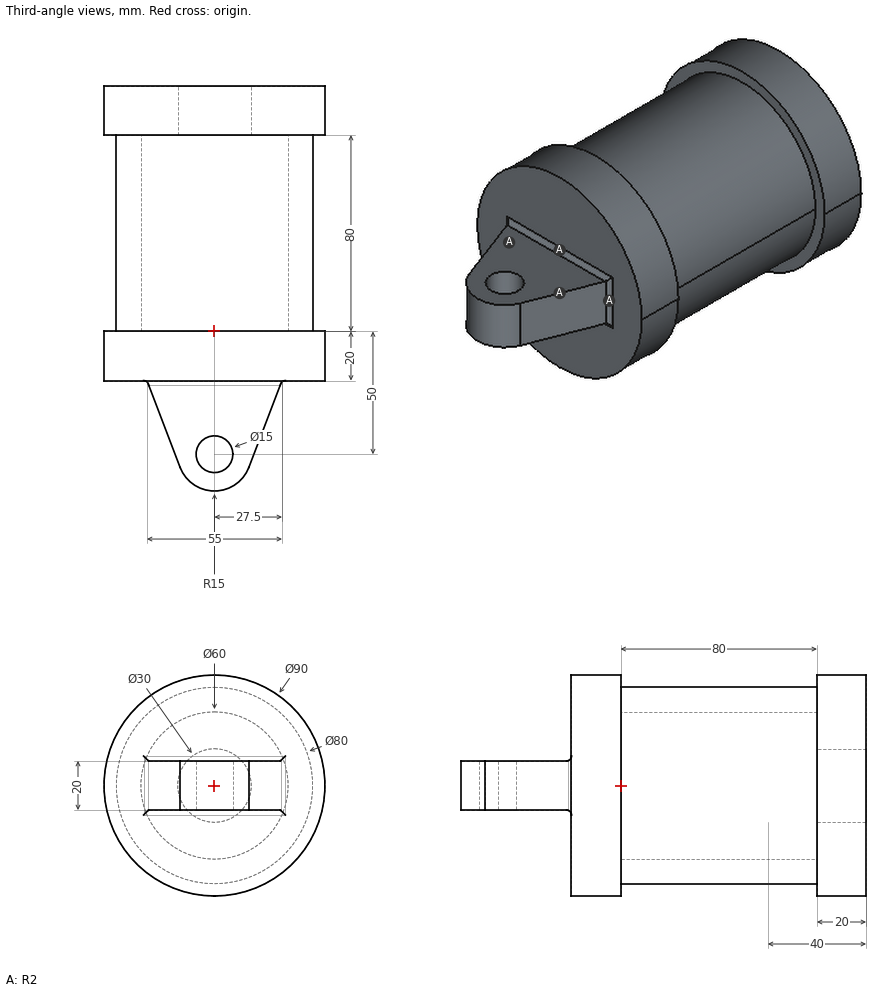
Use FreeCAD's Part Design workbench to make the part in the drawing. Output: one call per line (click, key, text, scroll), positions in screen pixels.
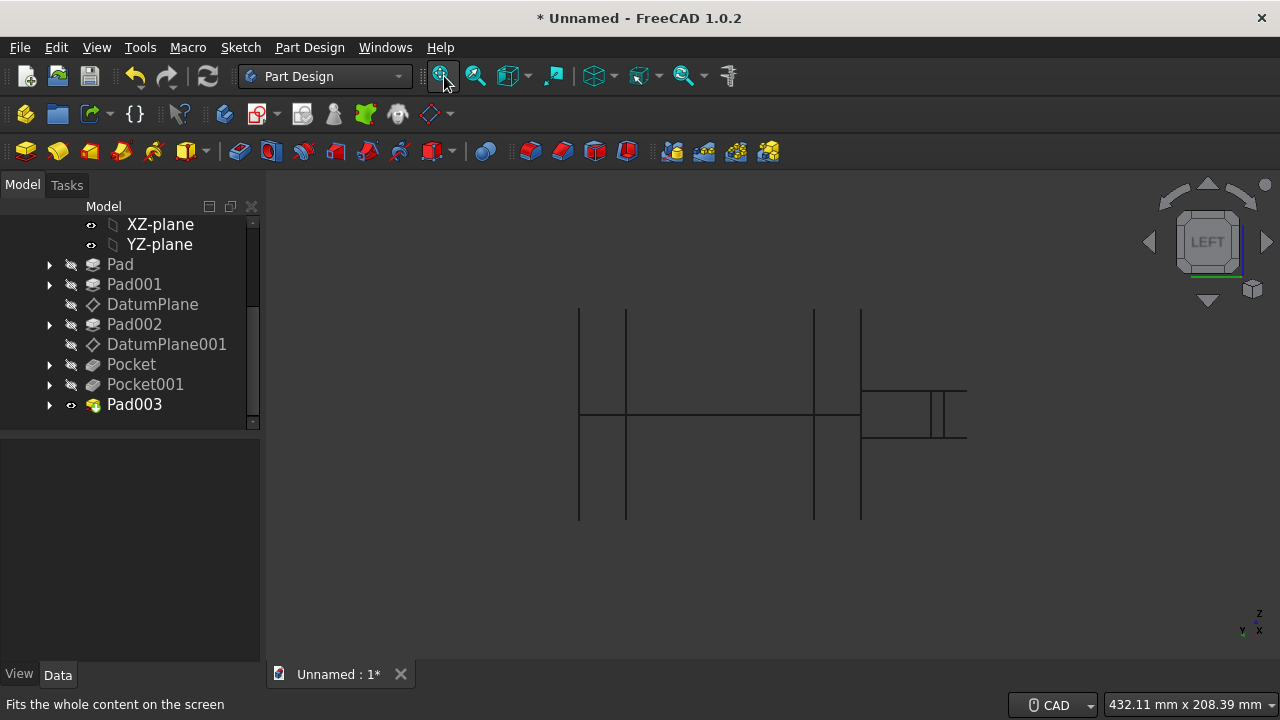
key(0)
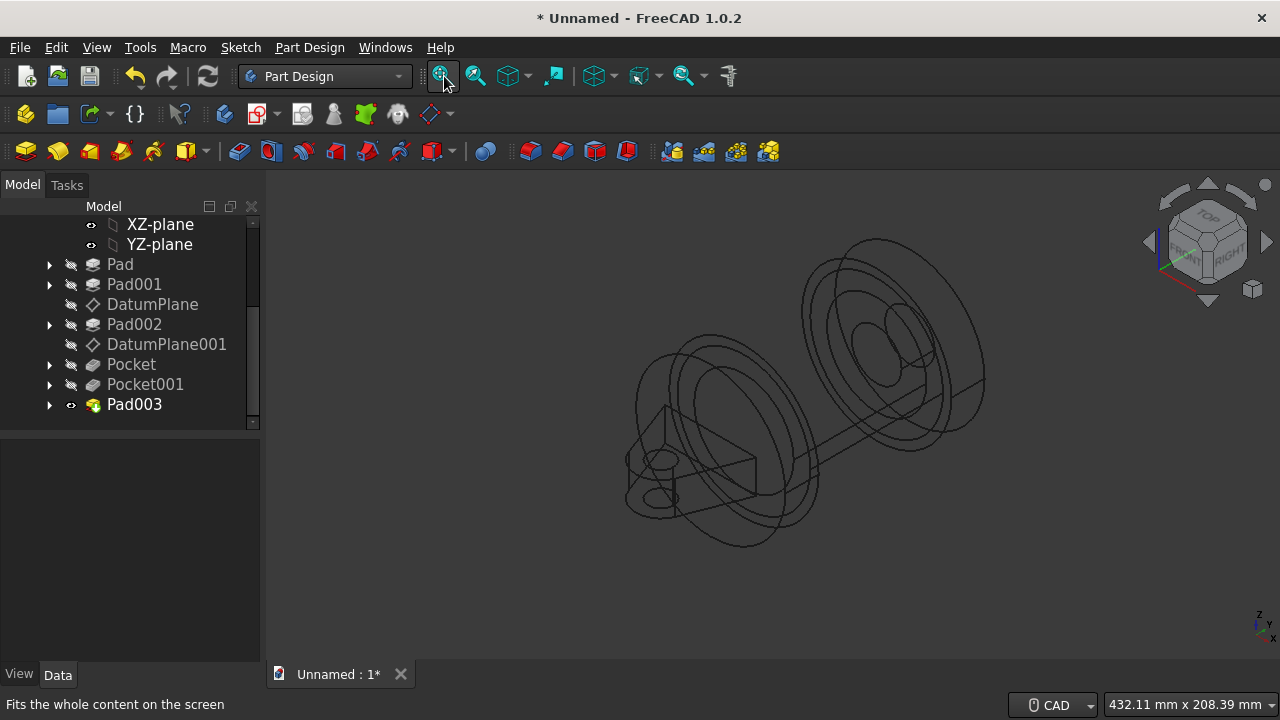
click(711, 430)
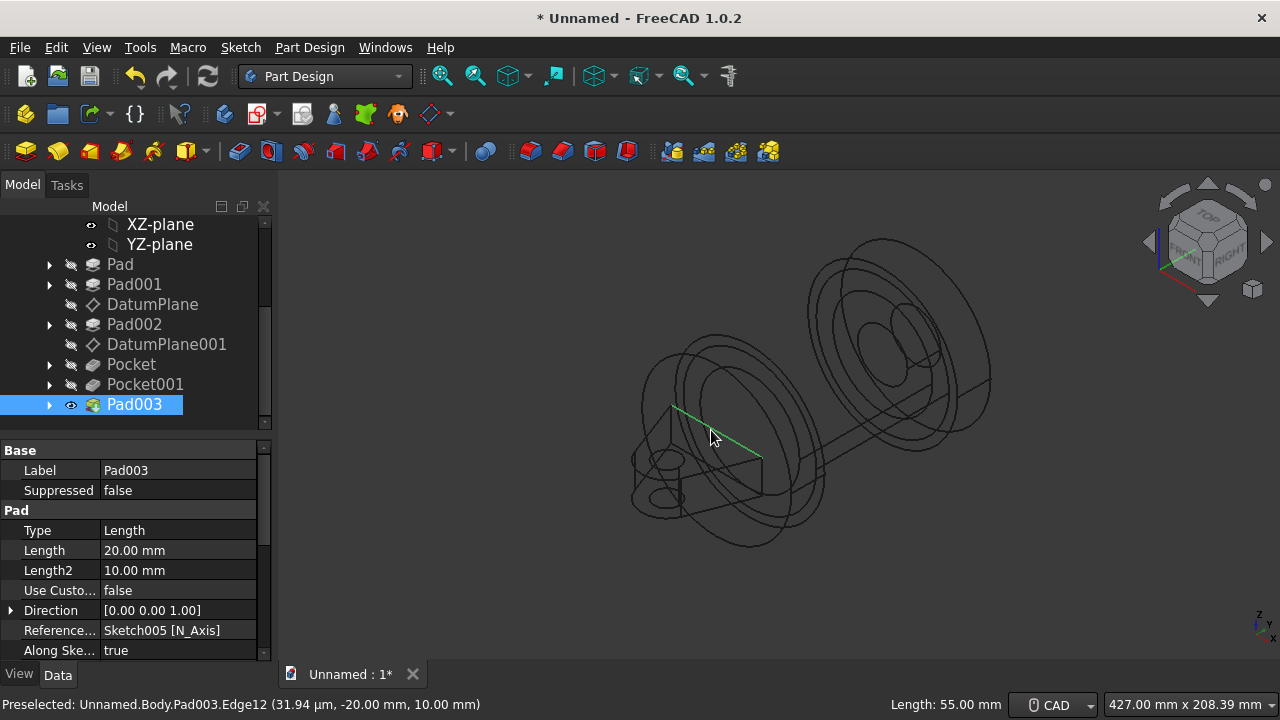
click(726, 474, ctrl)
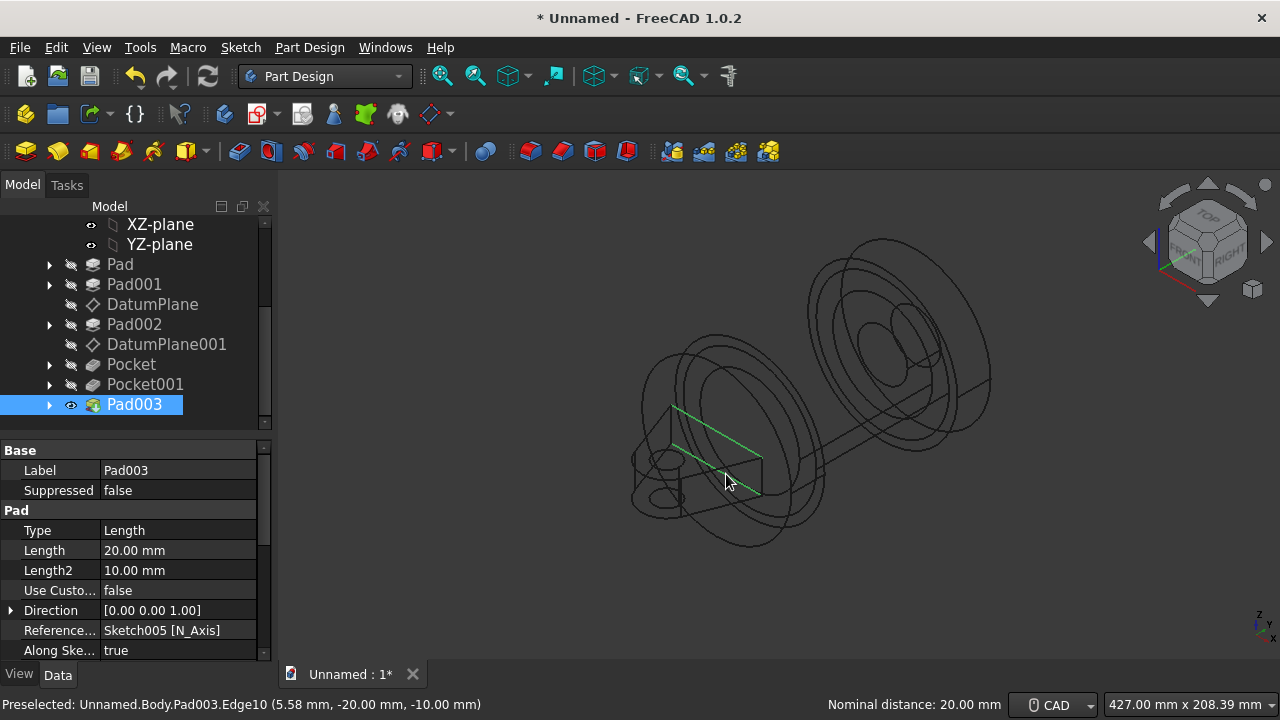
click(762, 476, ctrl)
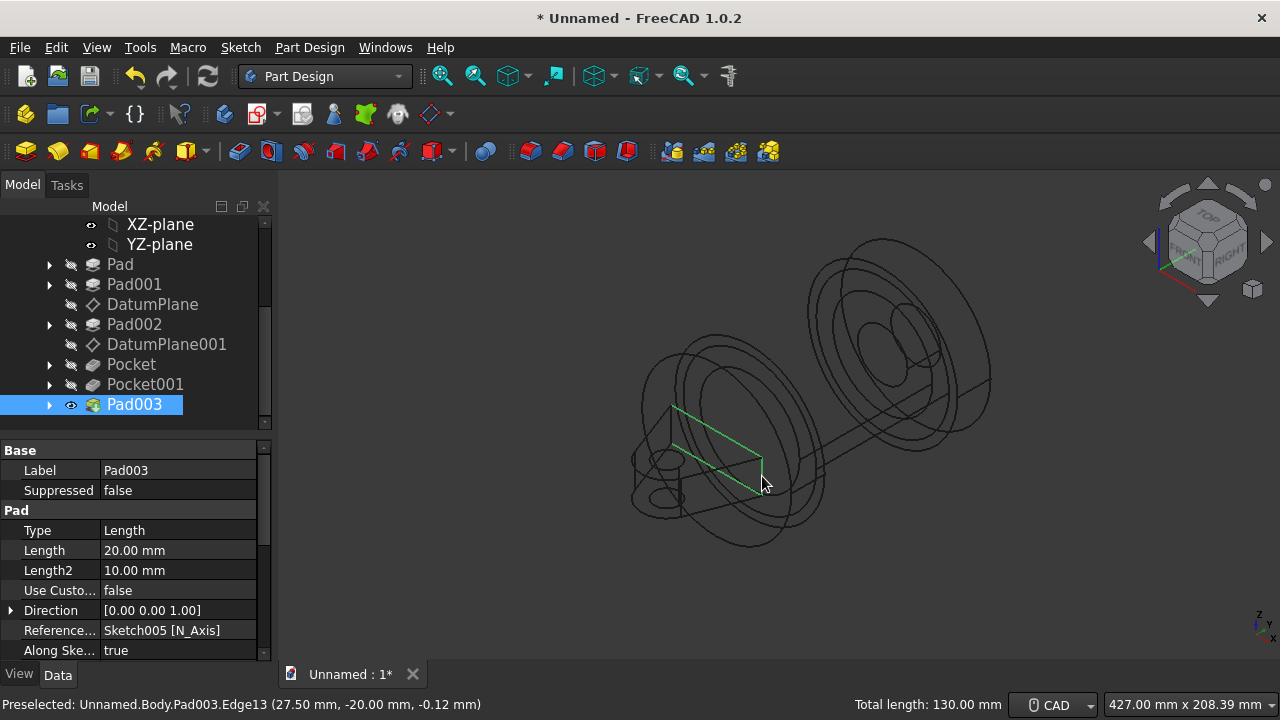
click(671, 423, ctrl)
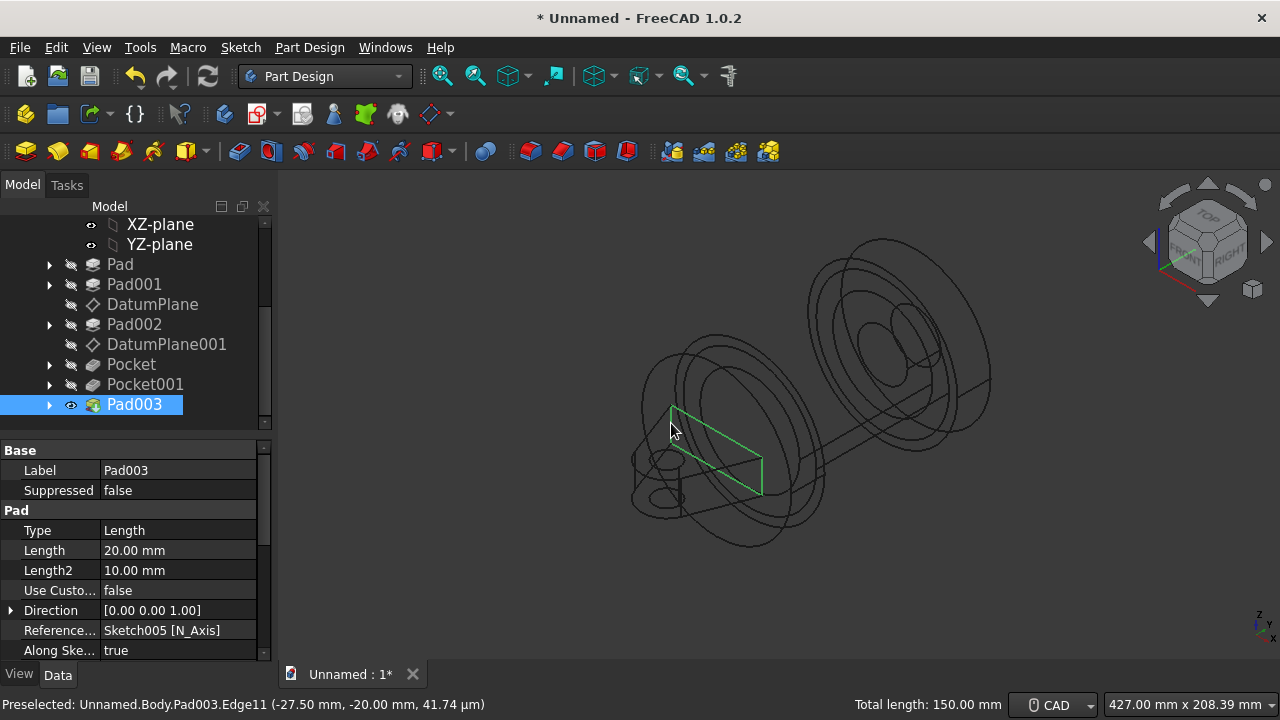
key(v)
key(1)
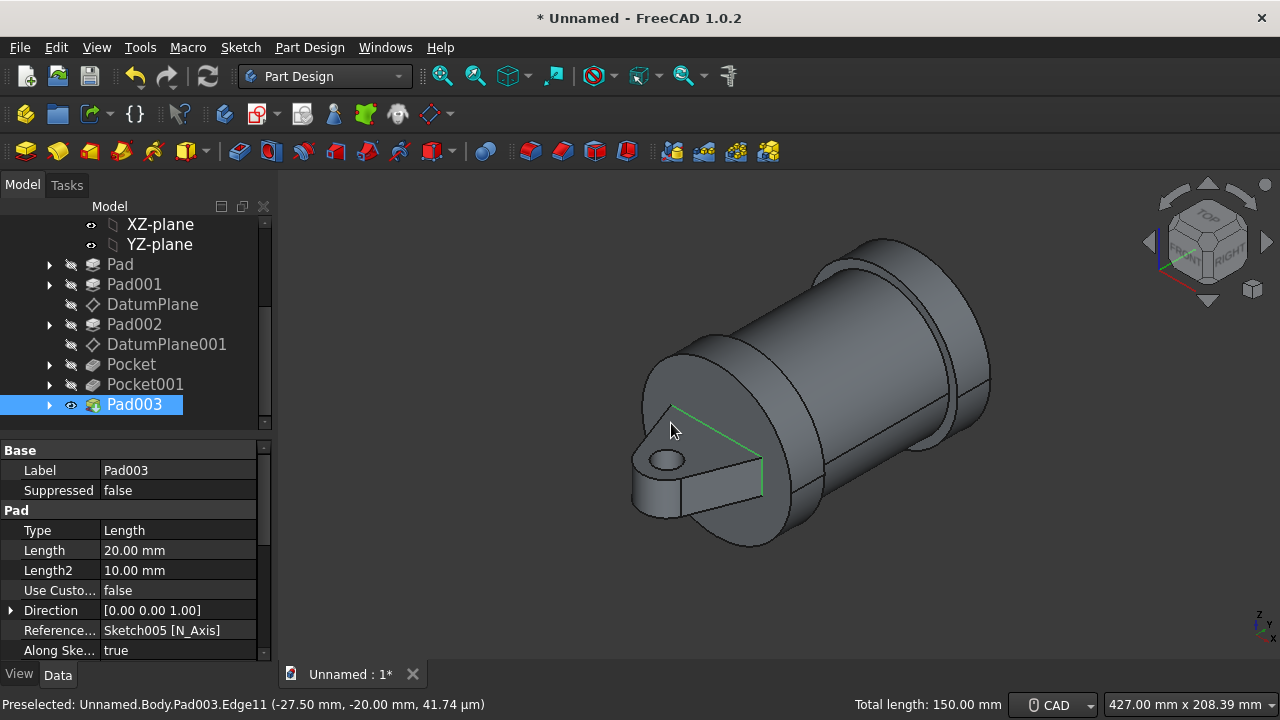
click(532, 152)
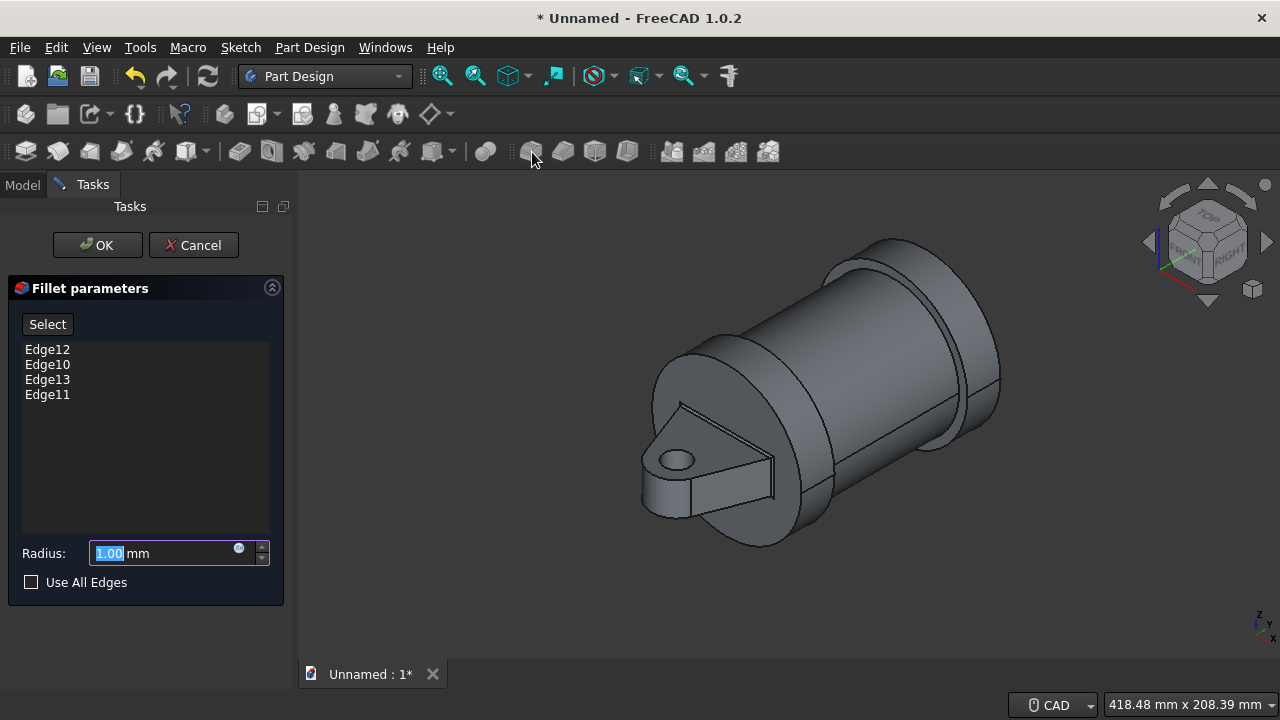
text(2)
key(Tab)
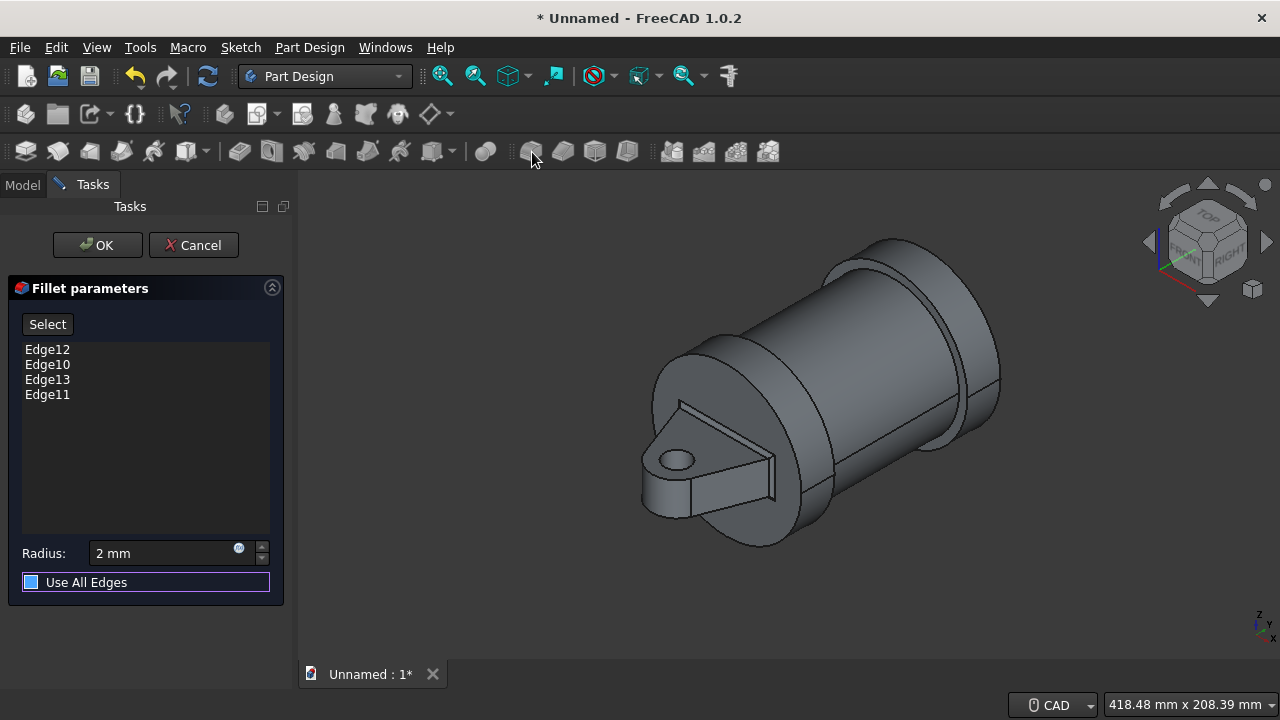
click(98, 245)